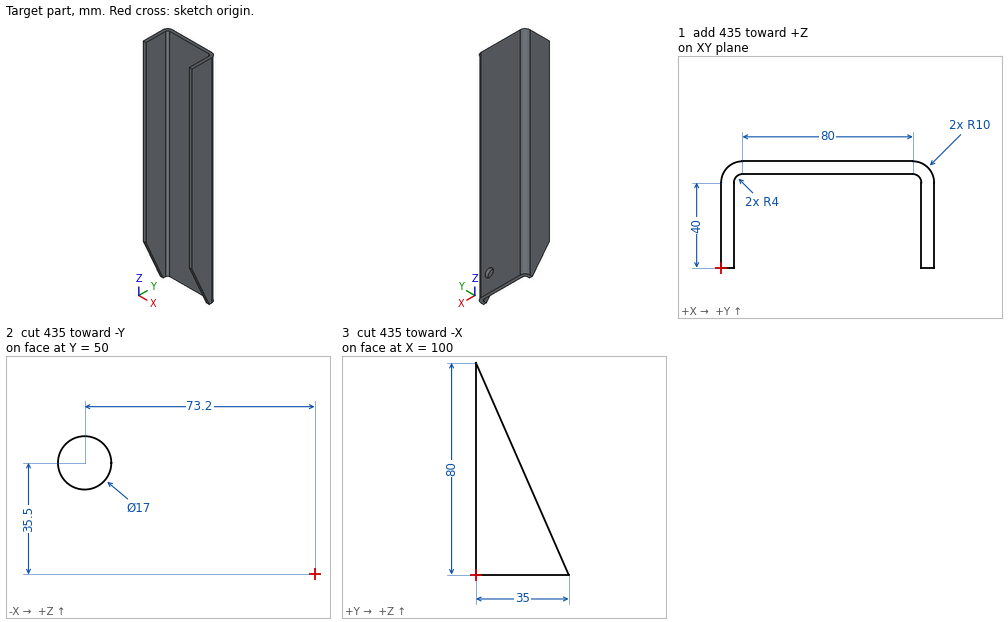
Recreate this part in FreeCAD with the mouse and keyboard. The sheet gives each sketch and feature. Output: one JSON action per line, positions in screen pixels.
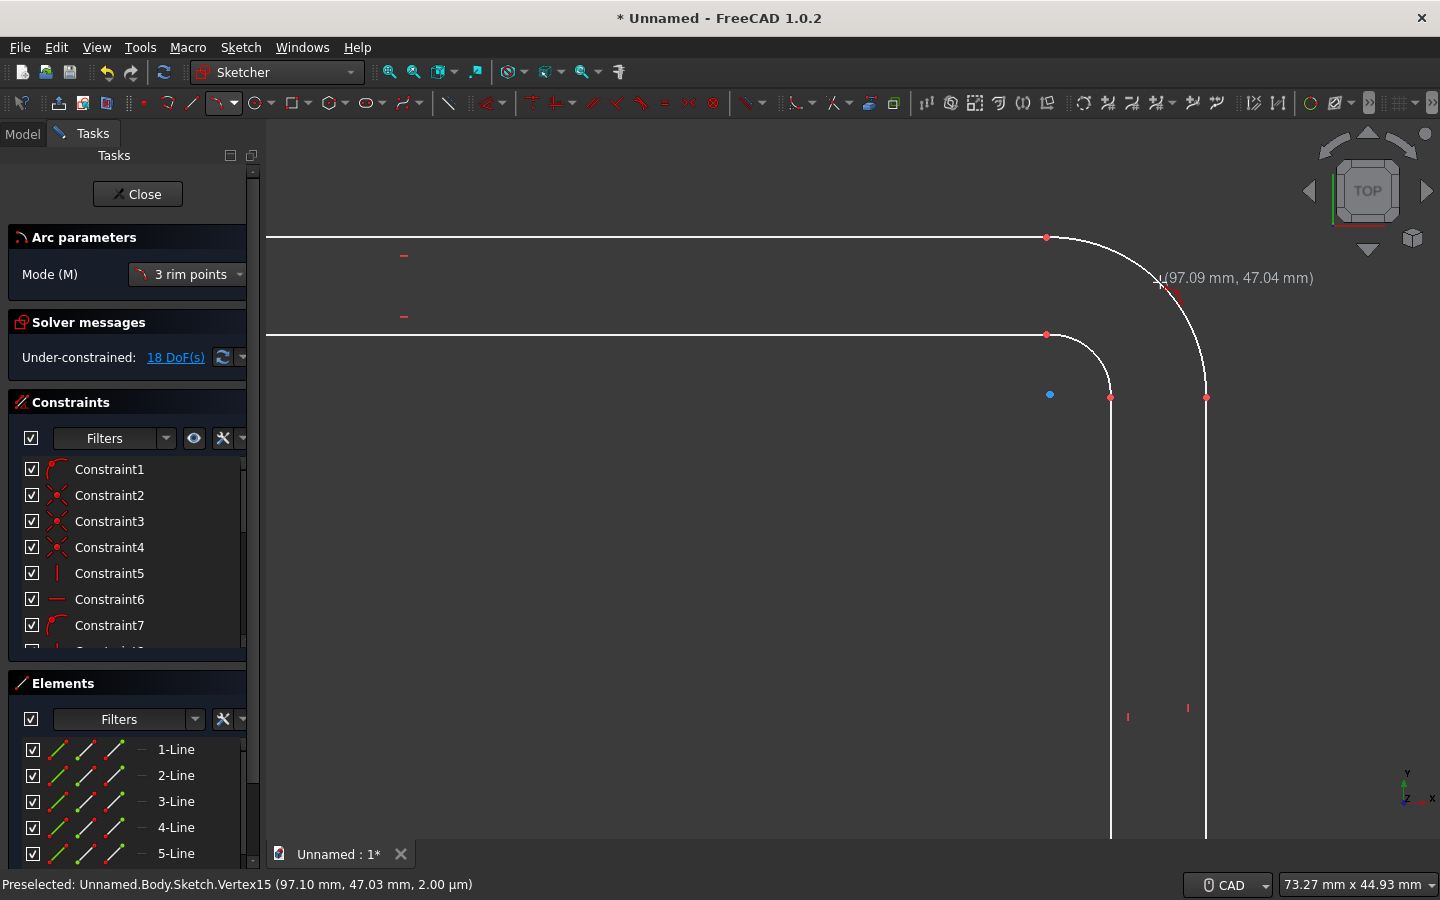
{"action": "scroll", "coordinate": [1094, 351], "scroll_direction": "down", "scroll_amount": 4}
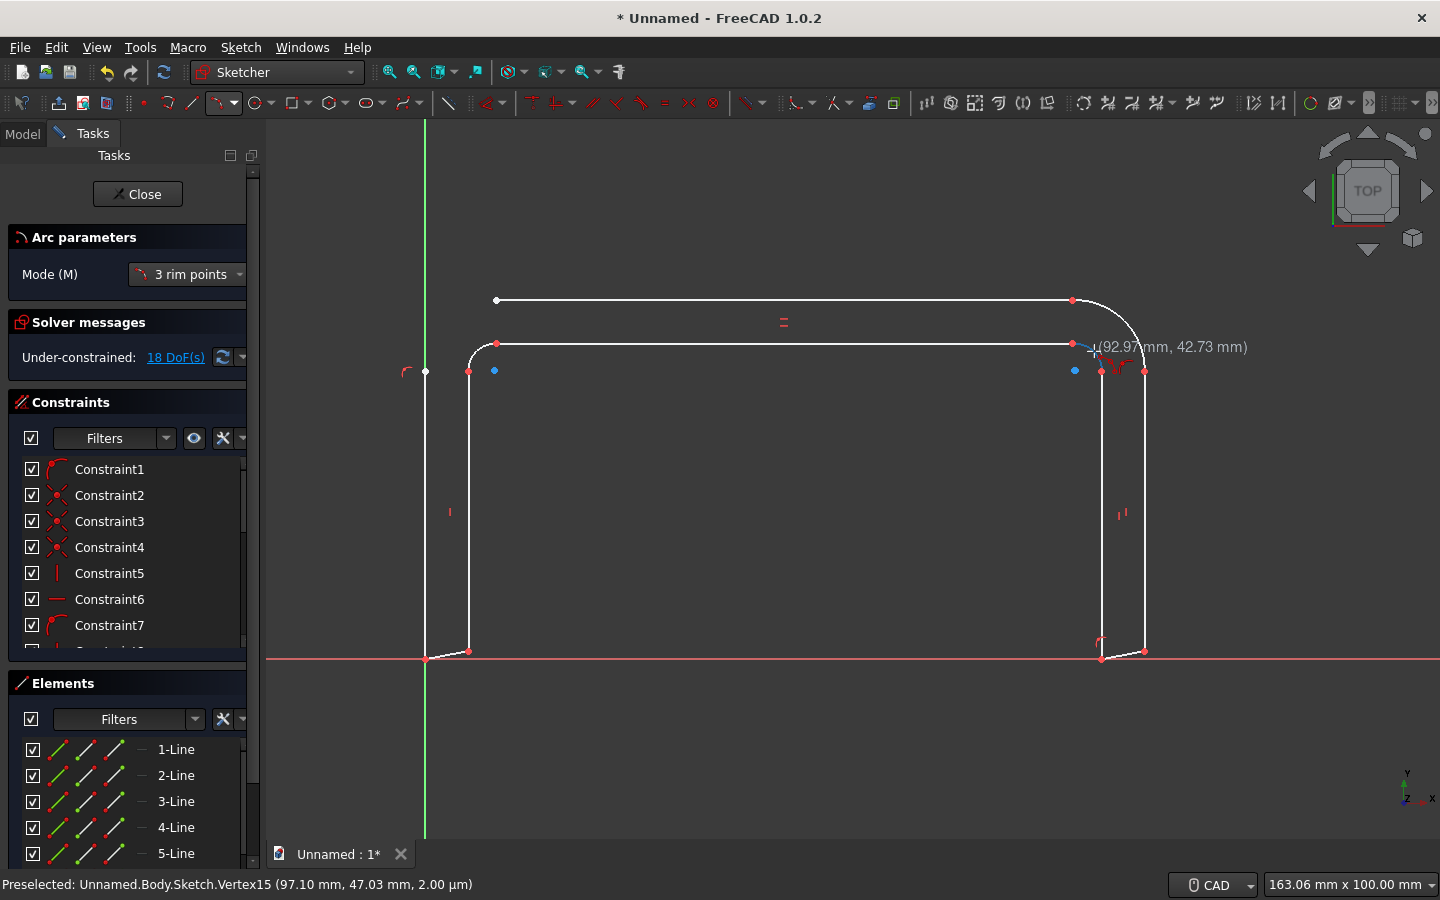
{"action": "left_click", "coordinate": [497, 300]}
{"action": "left_click", "coordinate": [425, 372]}
{"action": "left_click", "coordinate": [446, 320]}
{"action": "key", "text": "Escape"}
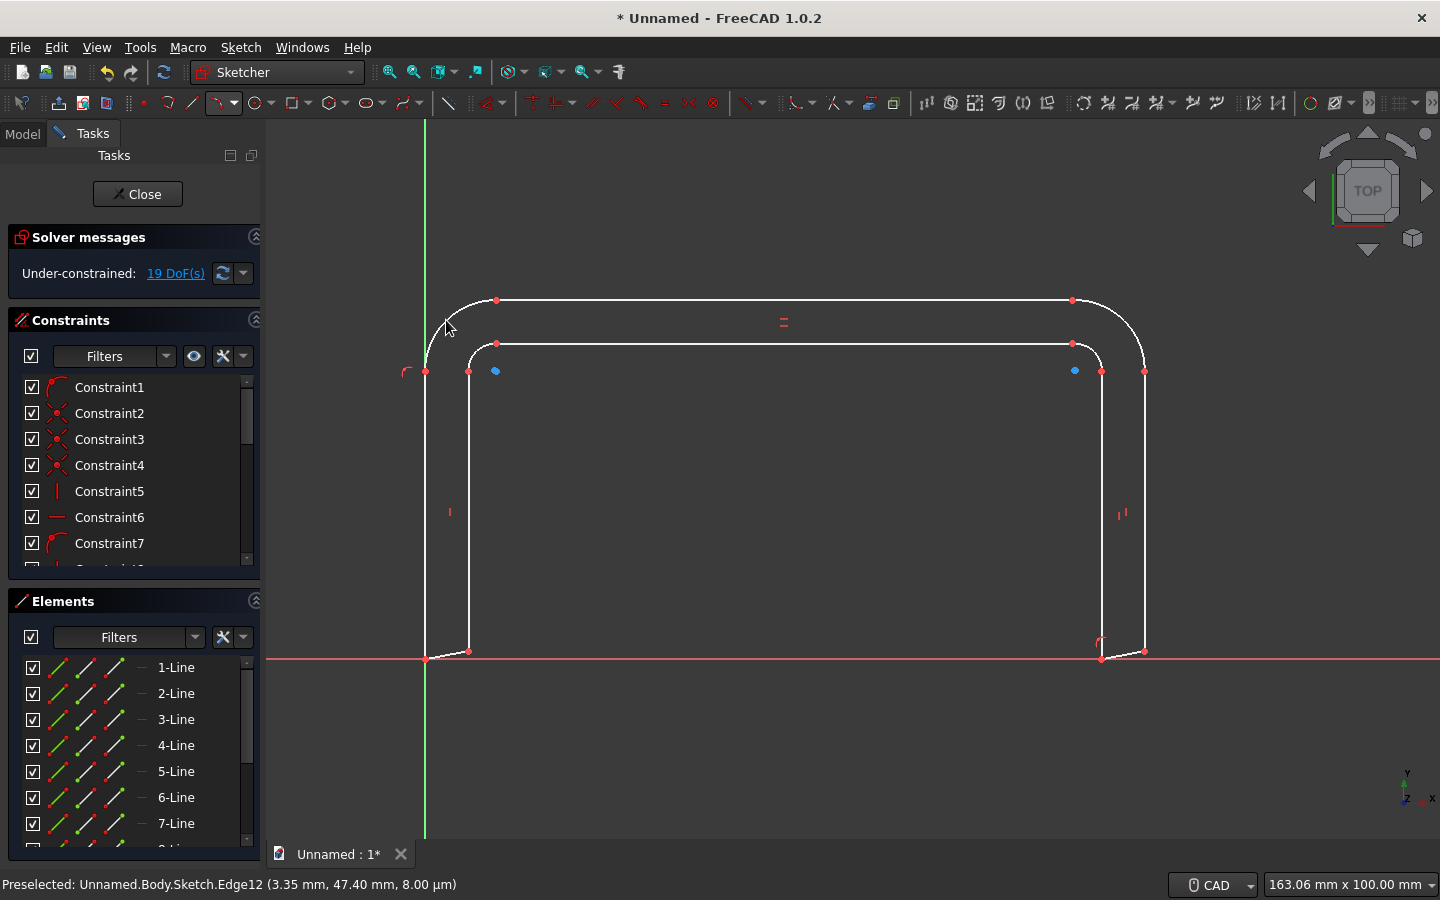
{"action": "left_click", "coordinate": [425, 458]}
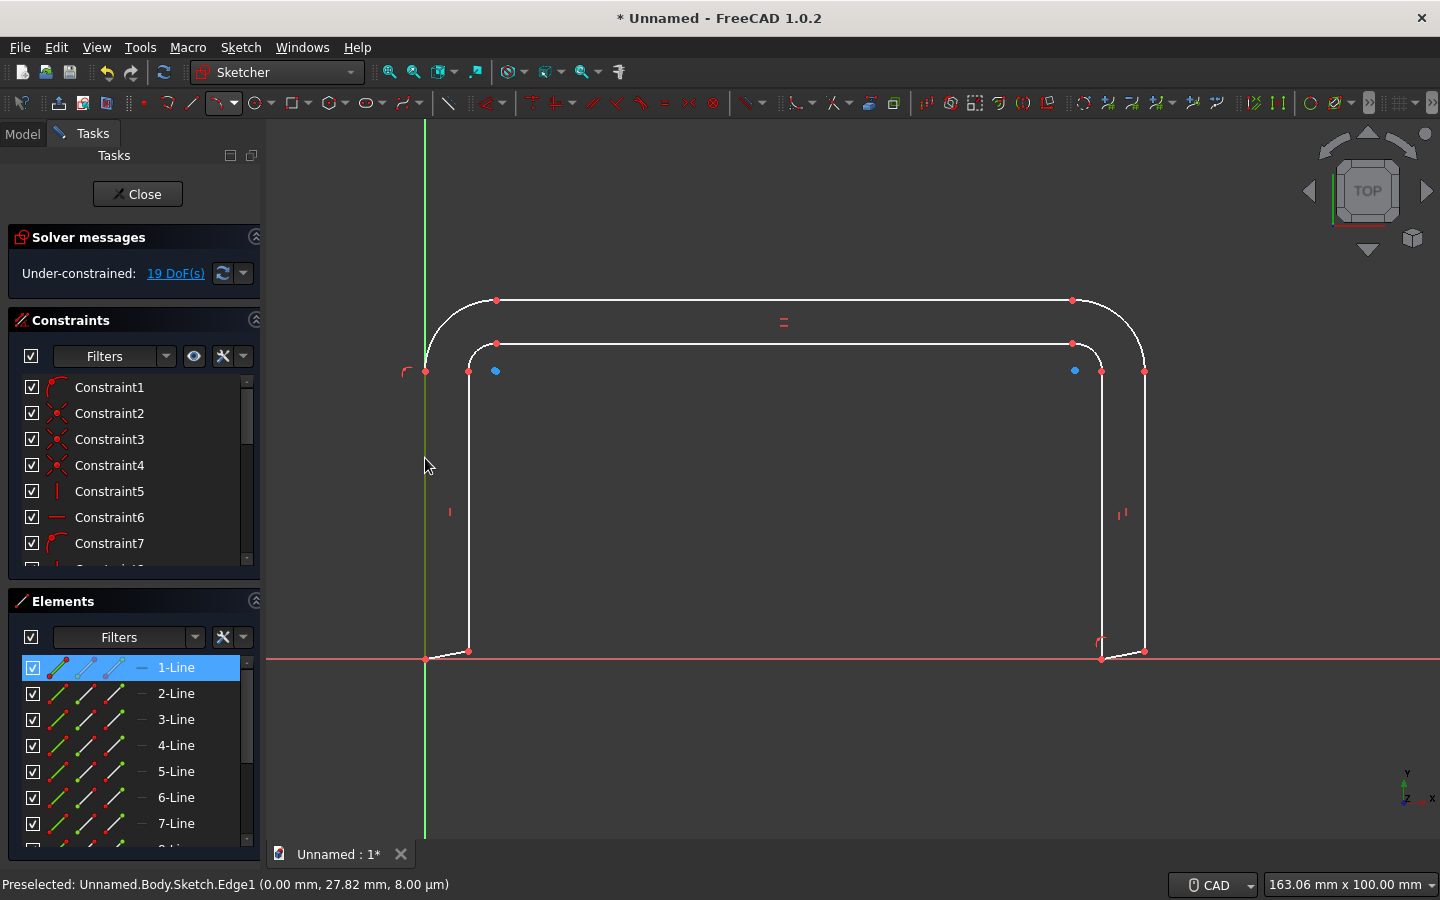
{"action": "left_click", "coordinate": [464, 308]}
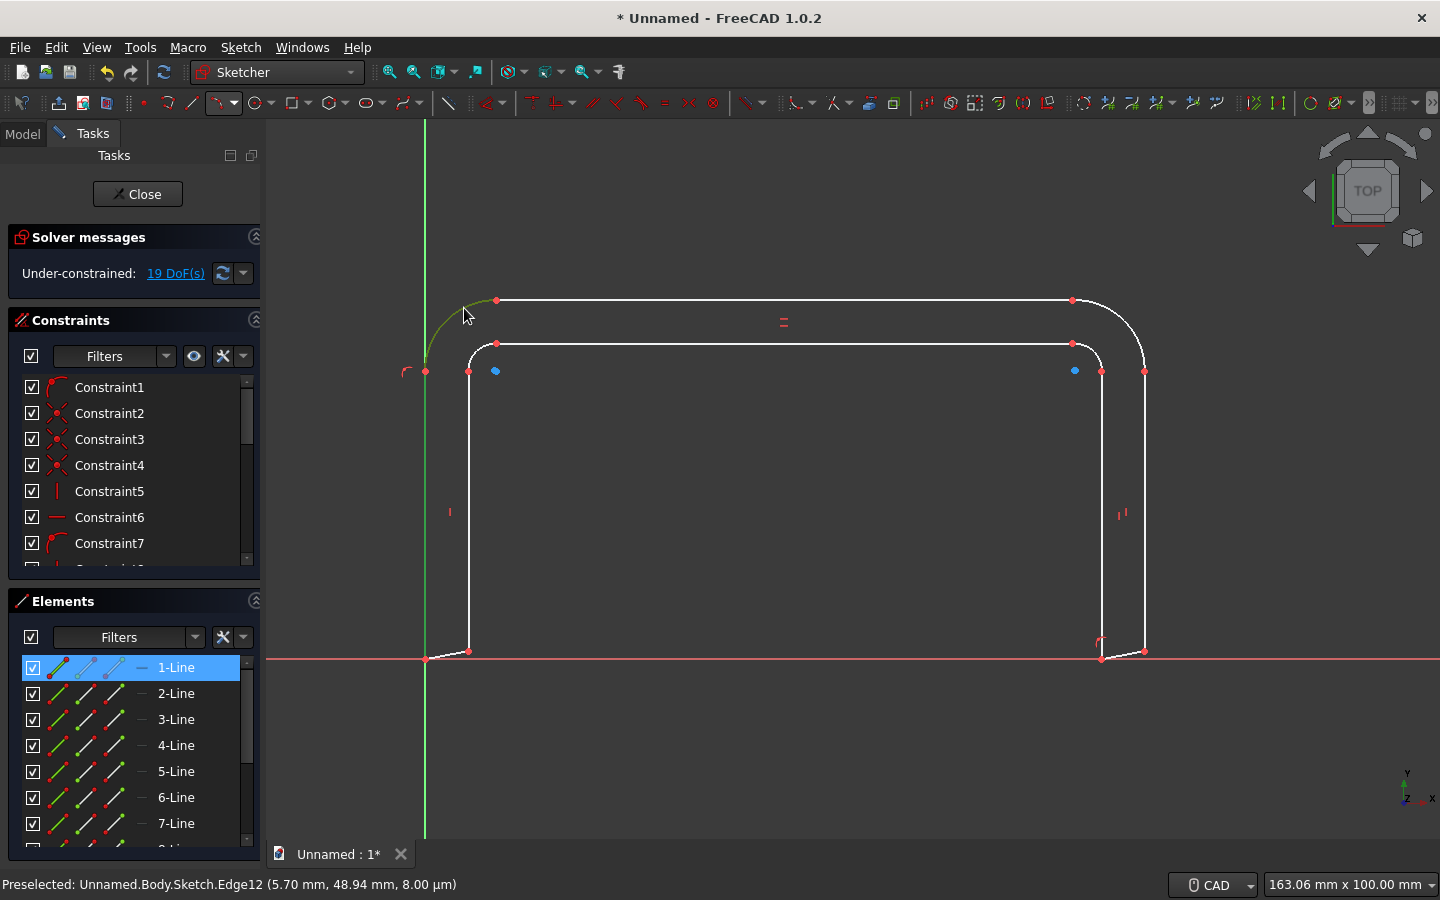
{"action": "left_click", "coordinate": [642, 104]}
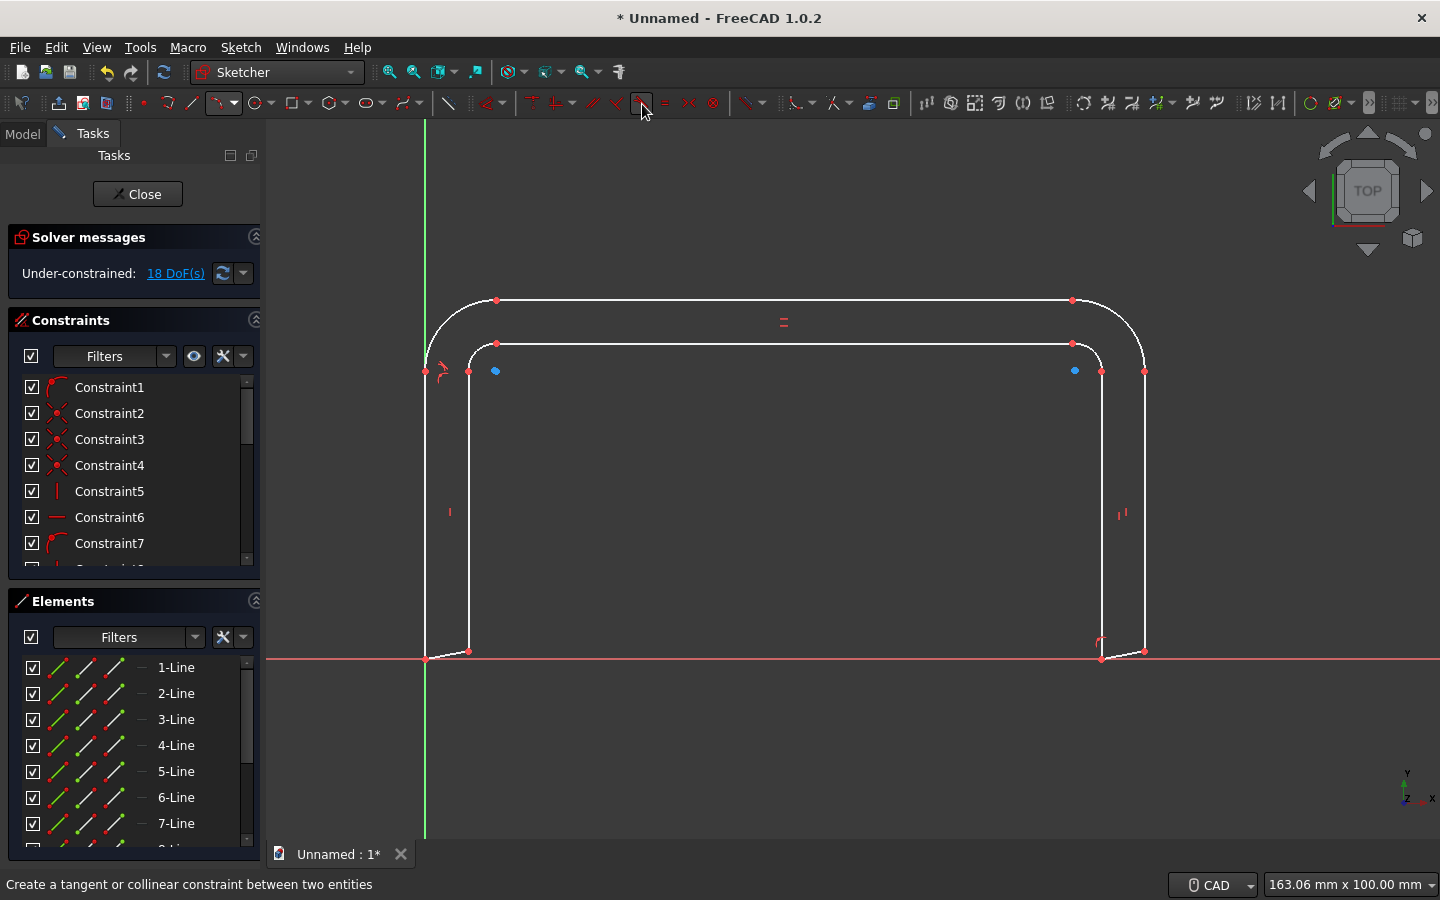
{"action": "left_click", "coordinate": [469, 567]}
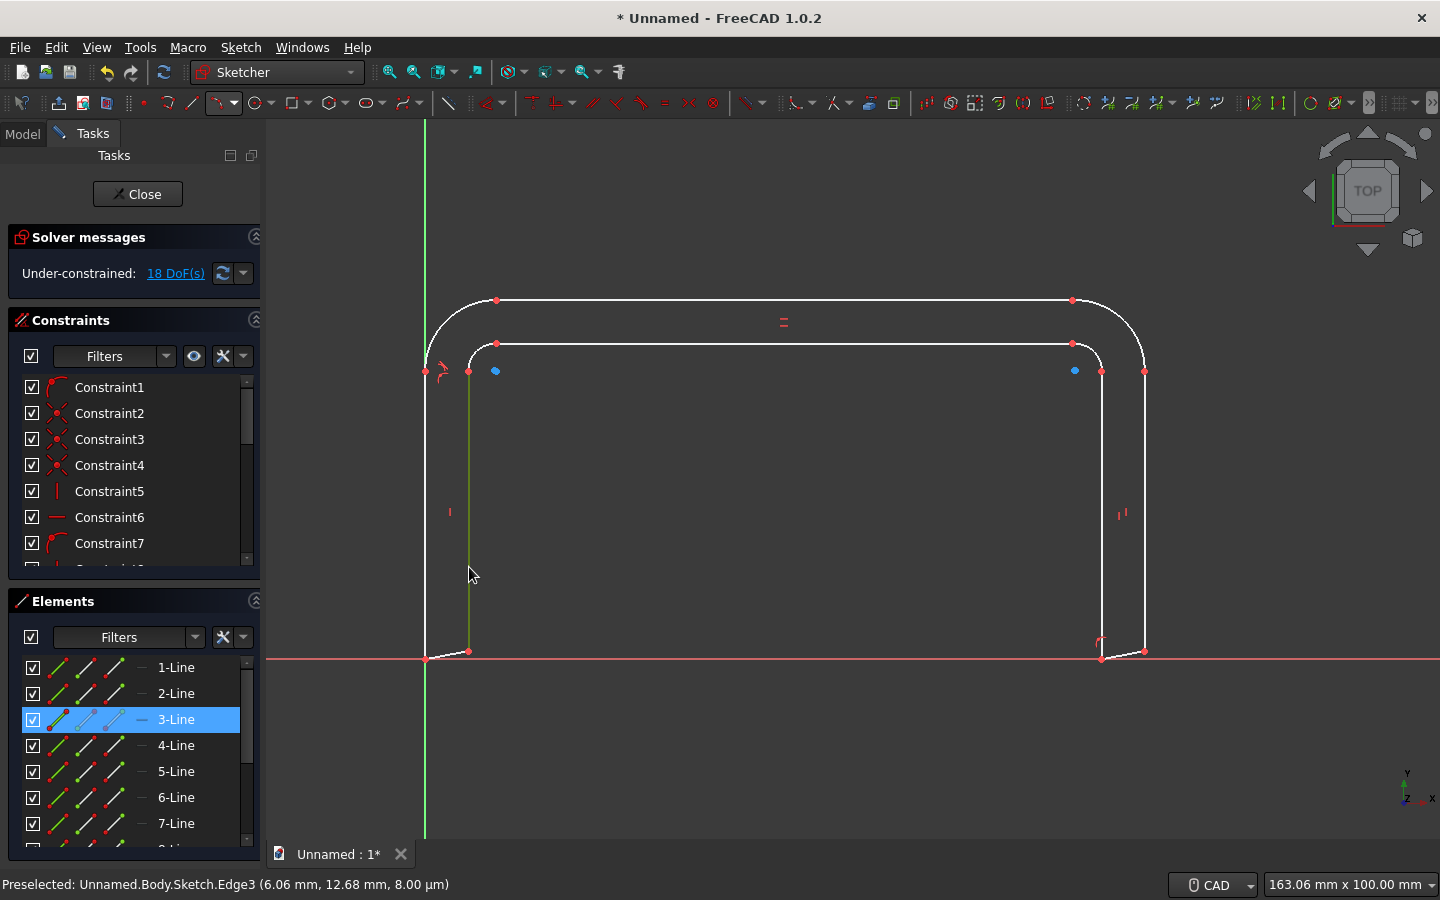
{"action": "left_click", "coordinate": [484, 346]}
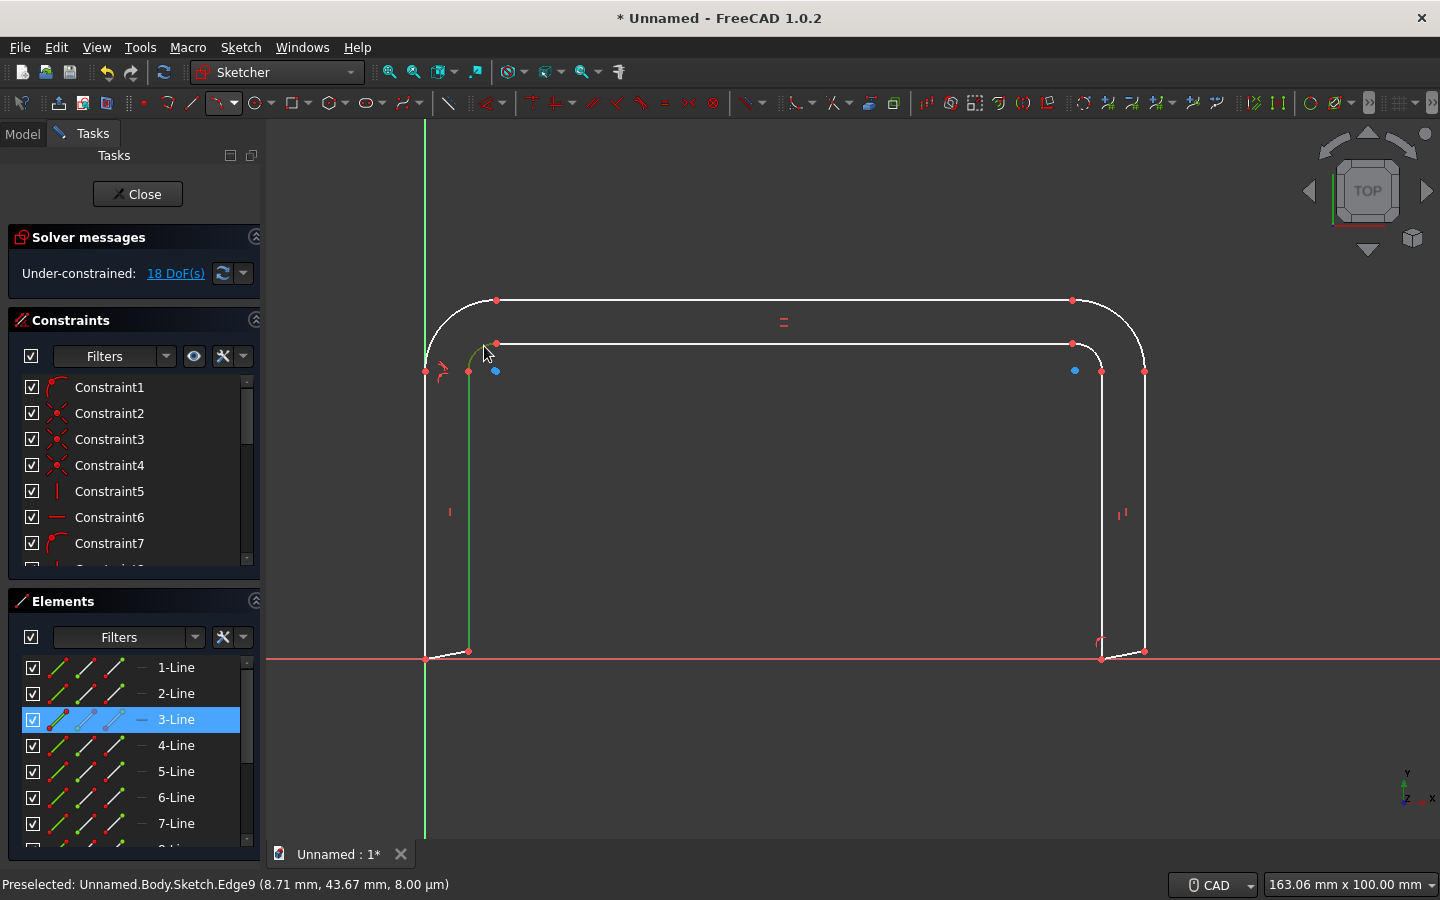
{"action": "left_click", "coordinate": [642, 104]}